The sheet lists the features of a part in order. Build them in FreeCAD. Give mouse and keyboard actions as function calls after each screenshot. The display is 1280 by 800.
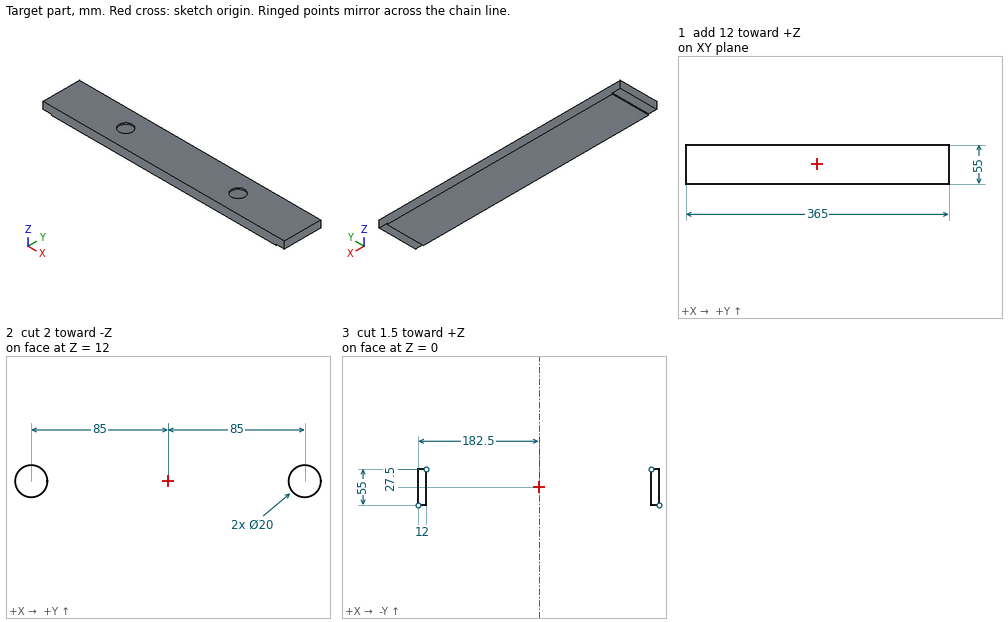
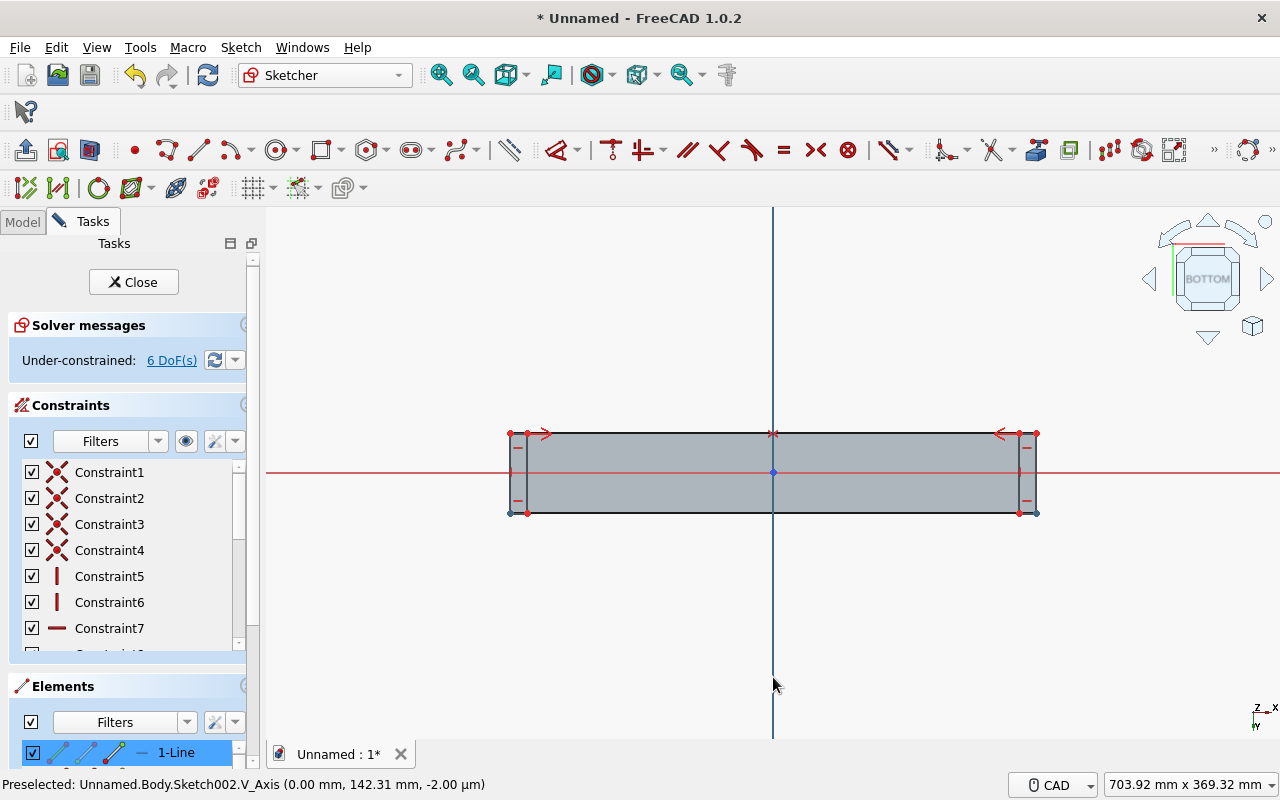
click(816, 150)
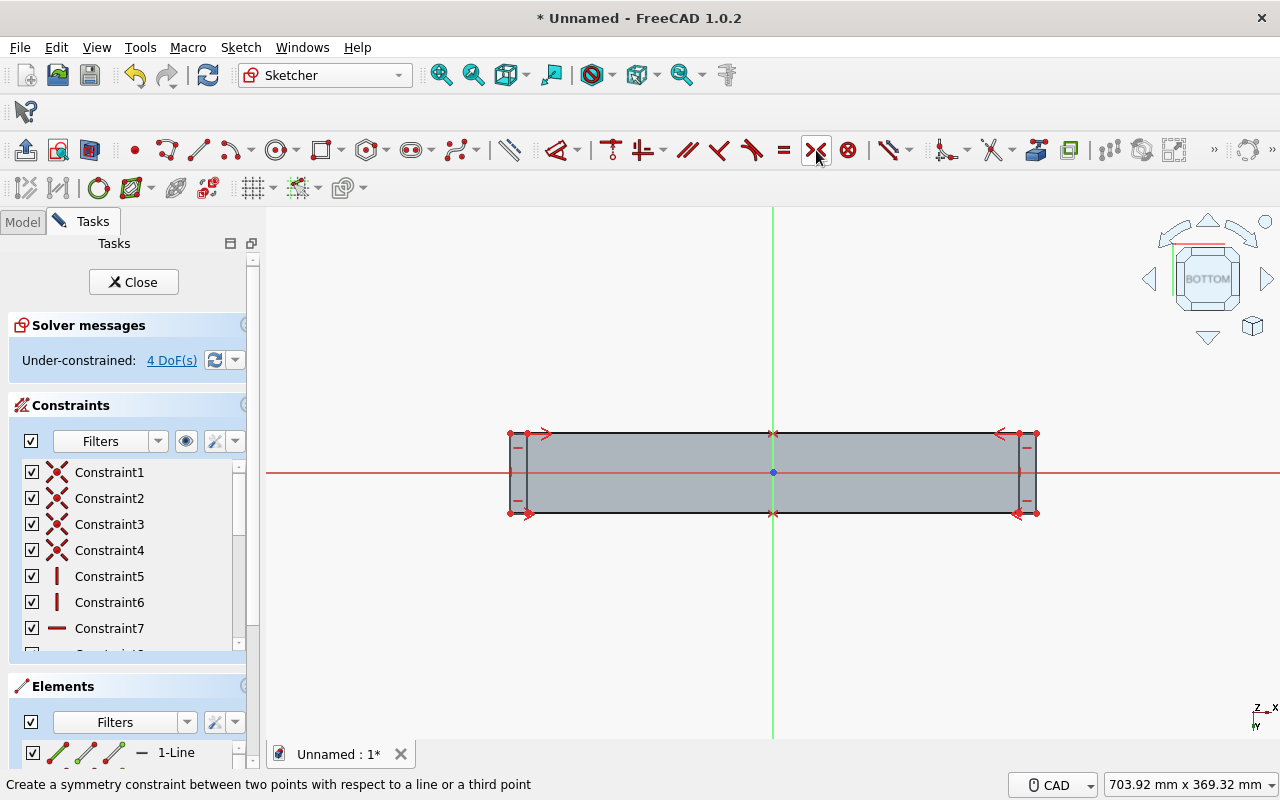
key(d)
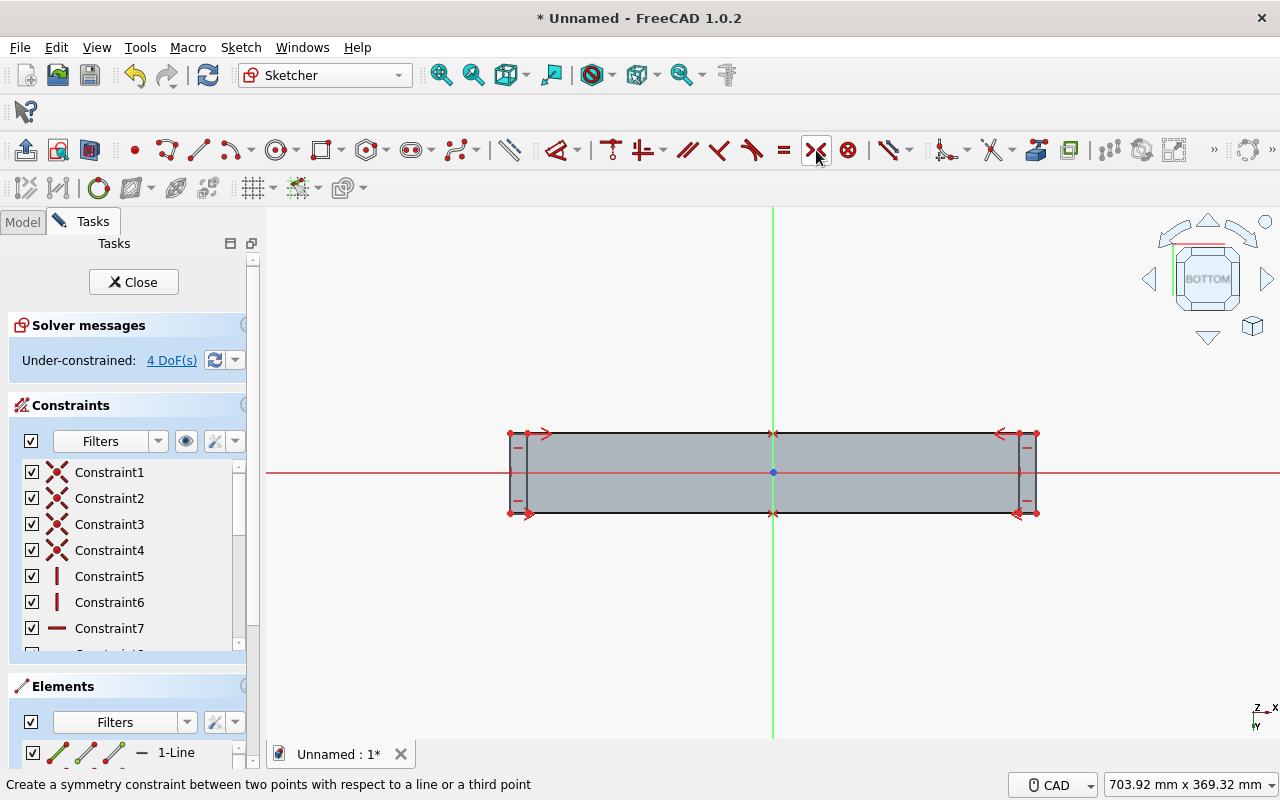
click(510, 458)
click(476, 456)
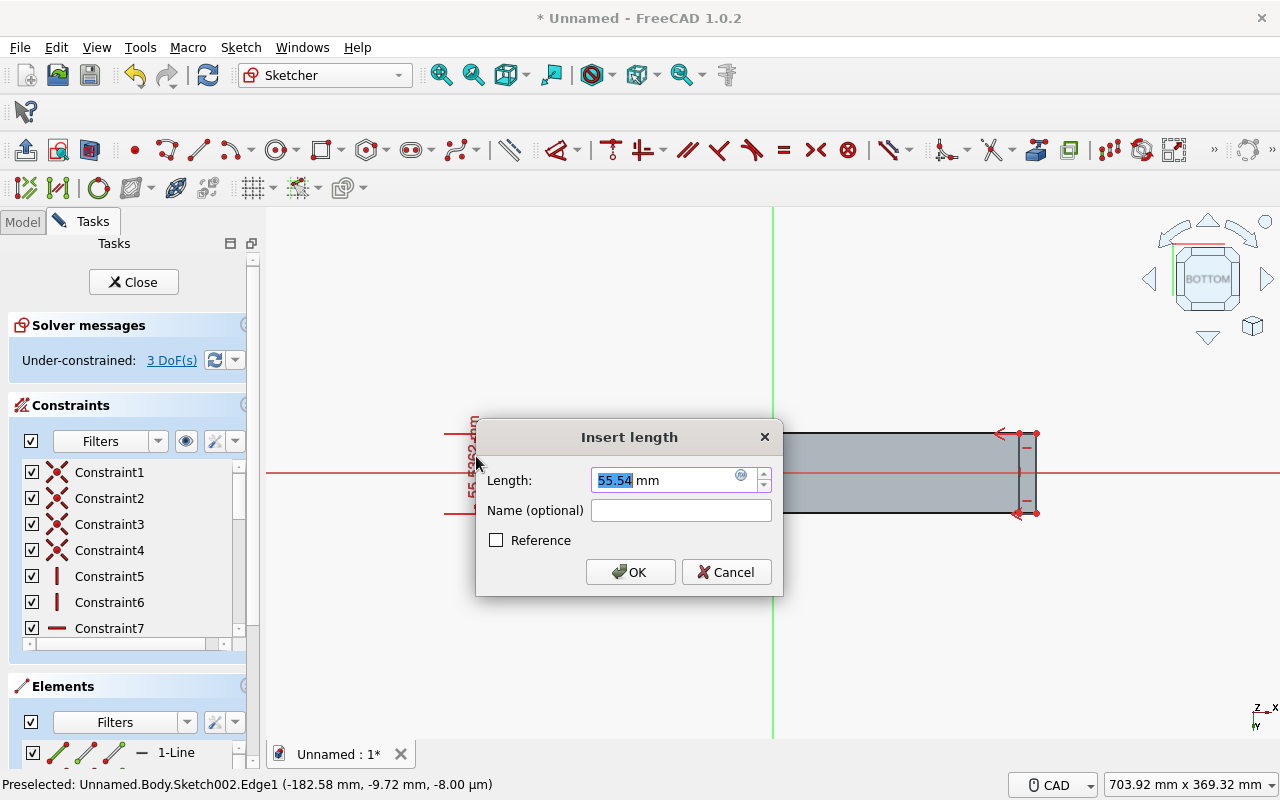
text(55)
key(Return)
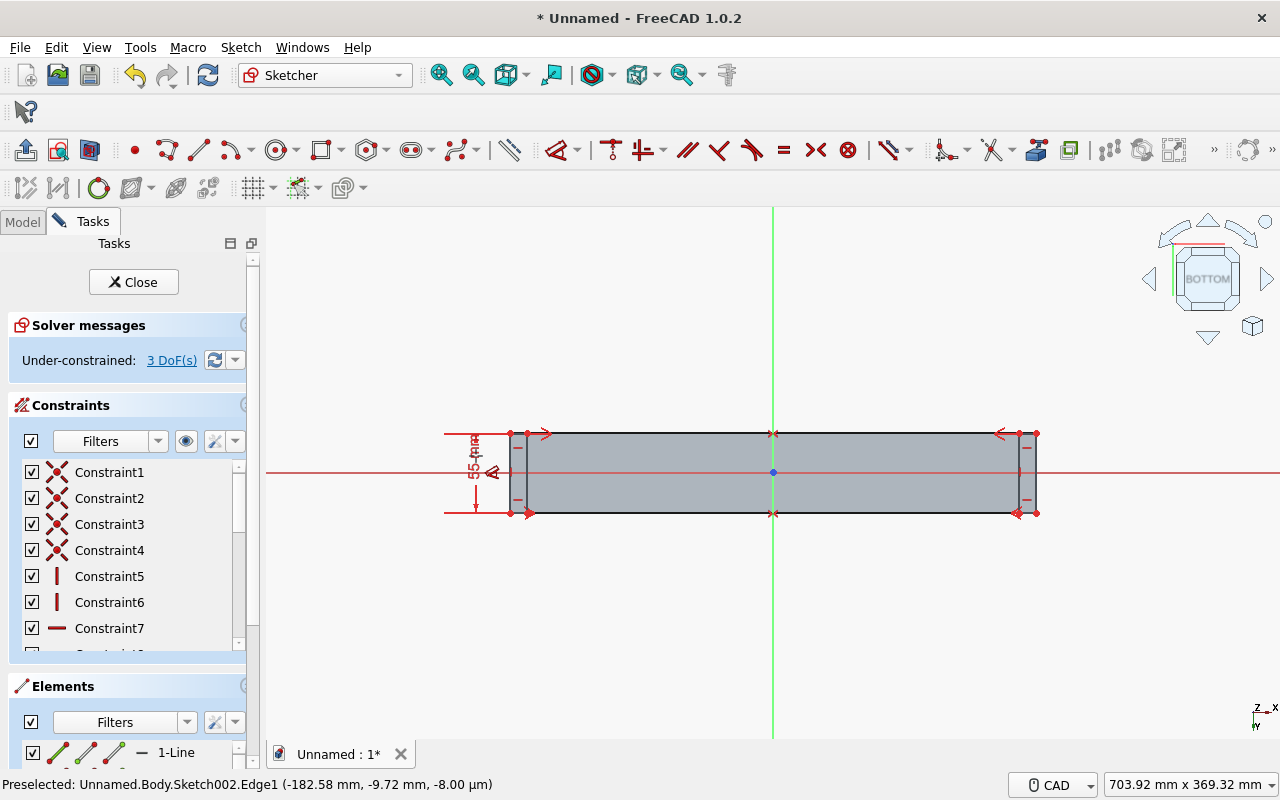
scroll(518, 513, up, 5)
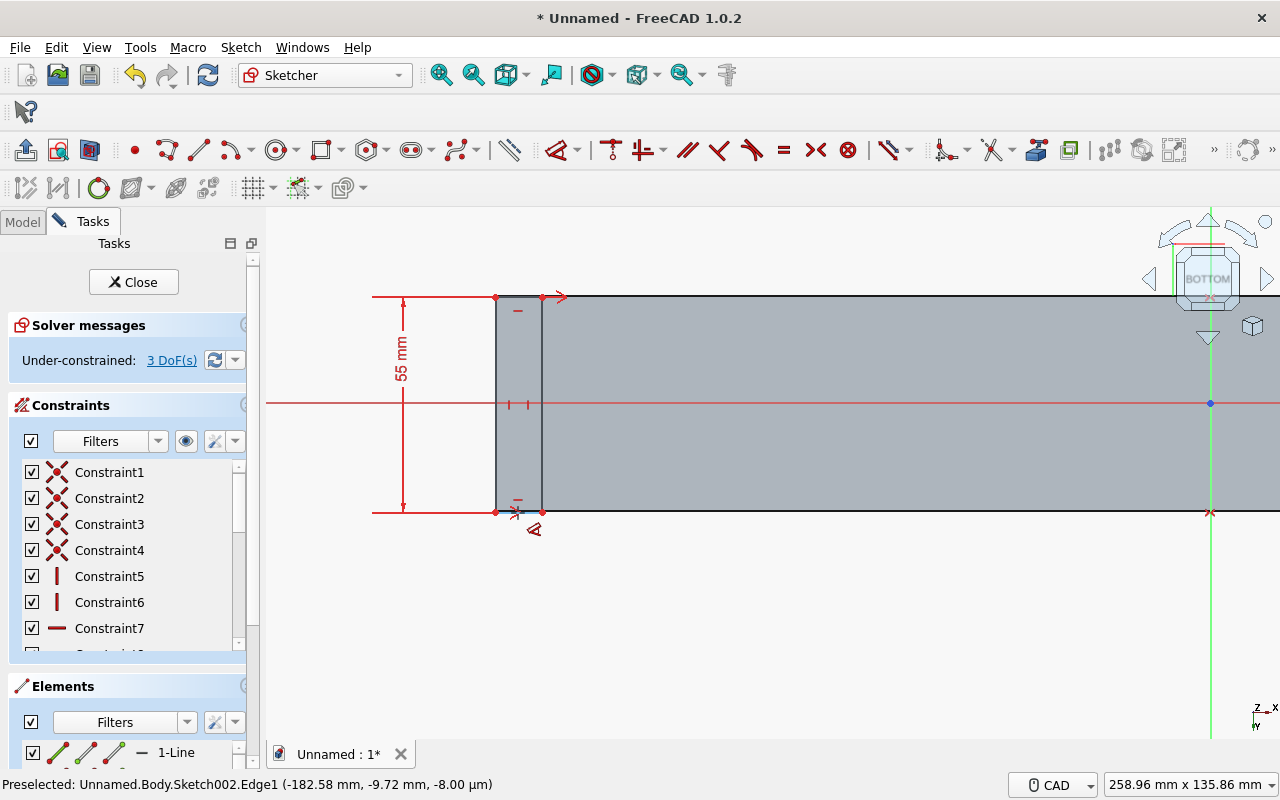
click(519, 513)
click(519, 547)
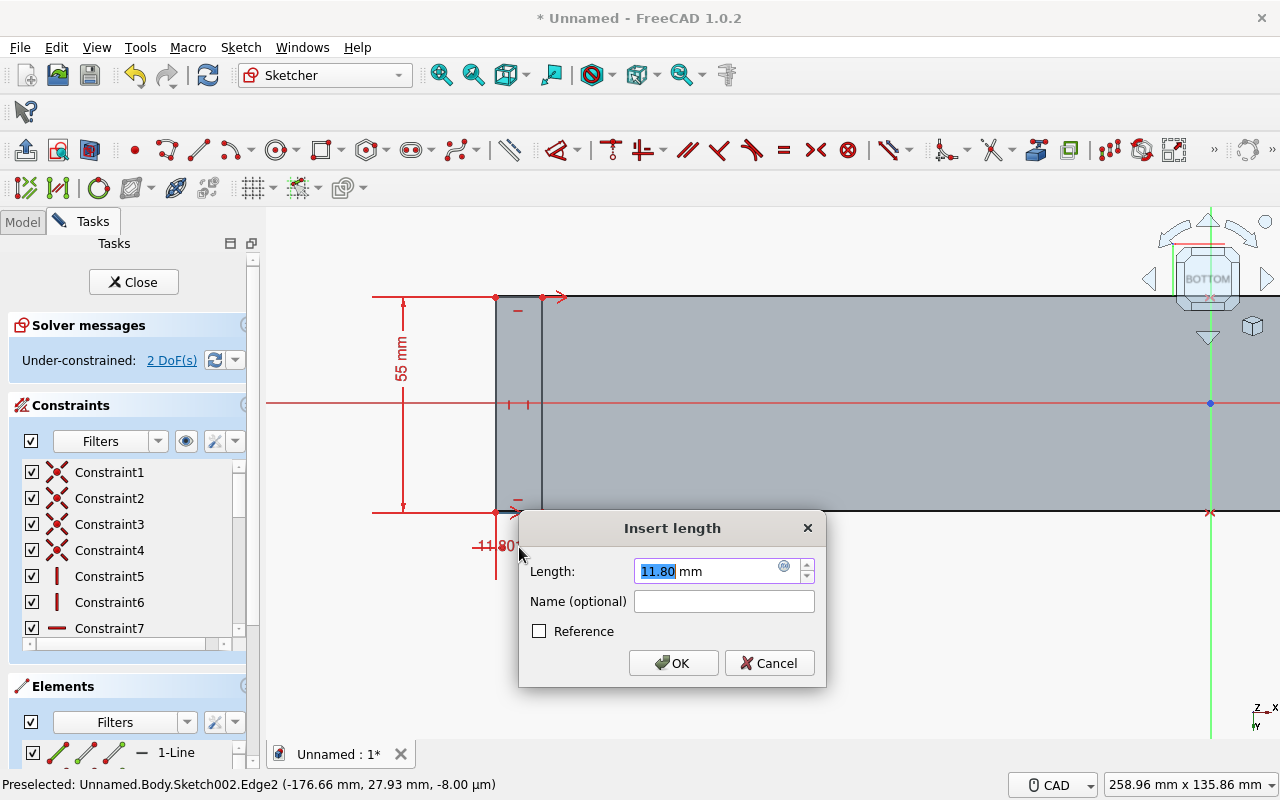
text(12)
key(Return)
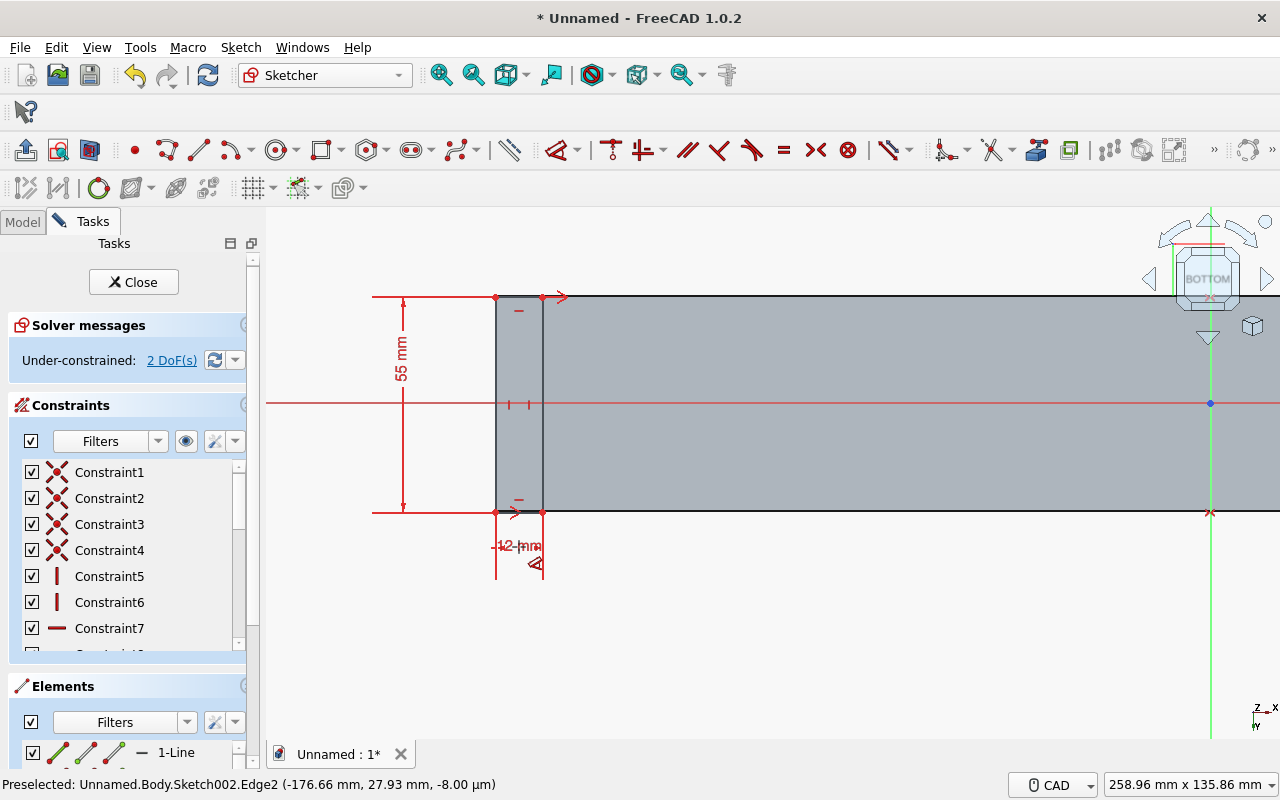
click(496, 297)
click(462, 326)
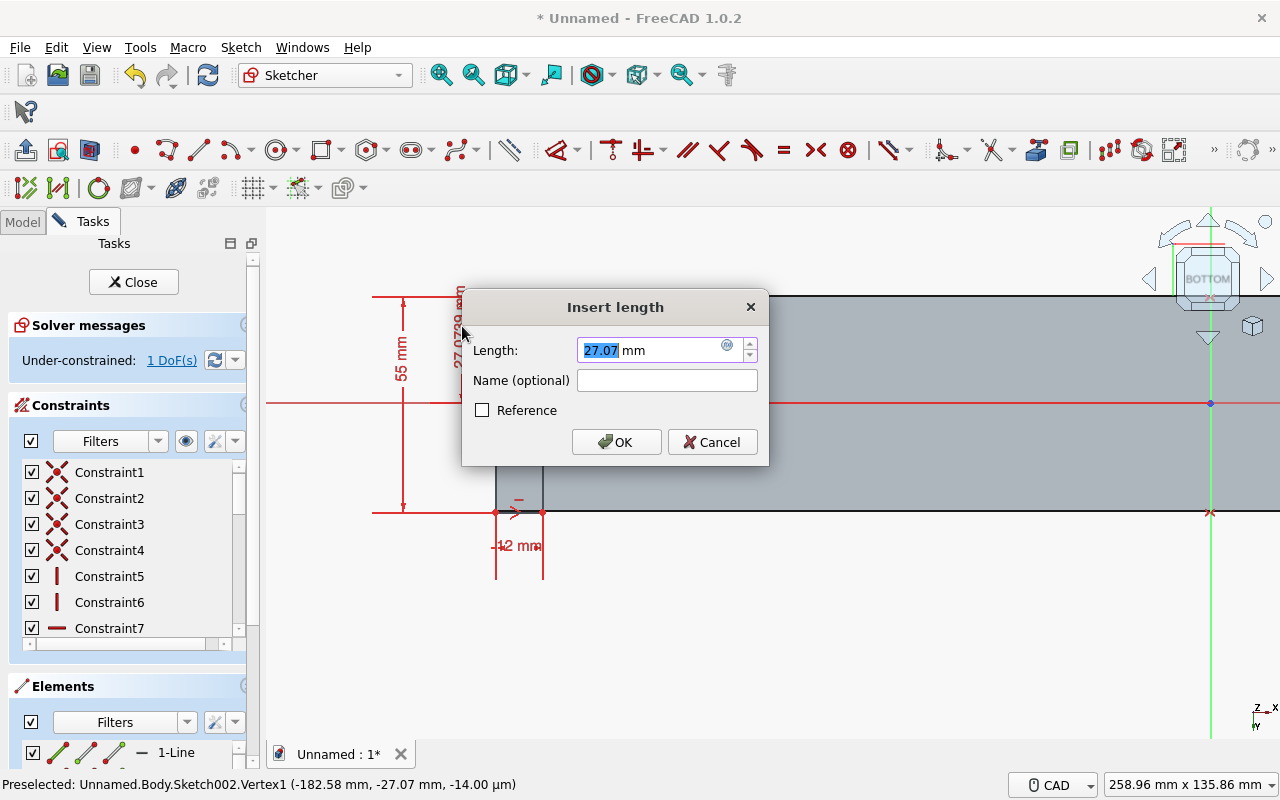
text(27.5)
key(Return)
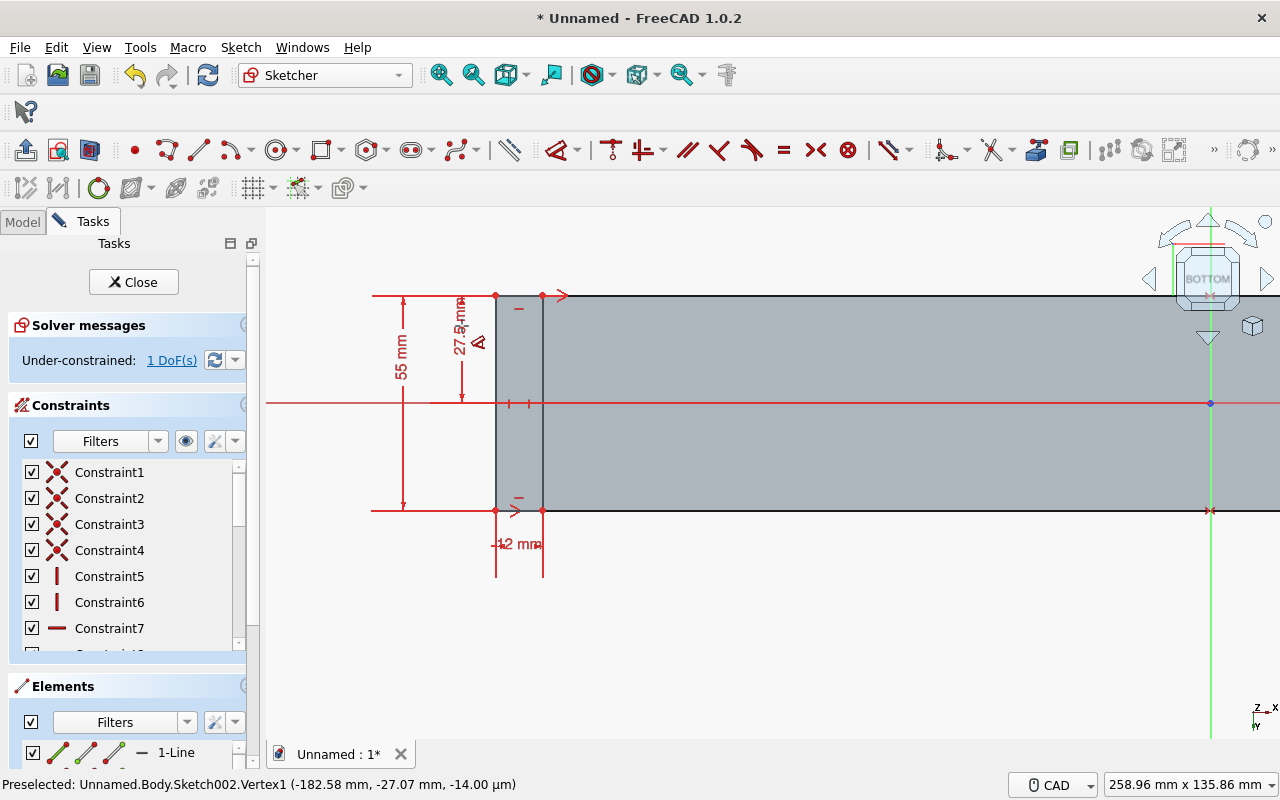
click(496, 296)
click(805, 262)